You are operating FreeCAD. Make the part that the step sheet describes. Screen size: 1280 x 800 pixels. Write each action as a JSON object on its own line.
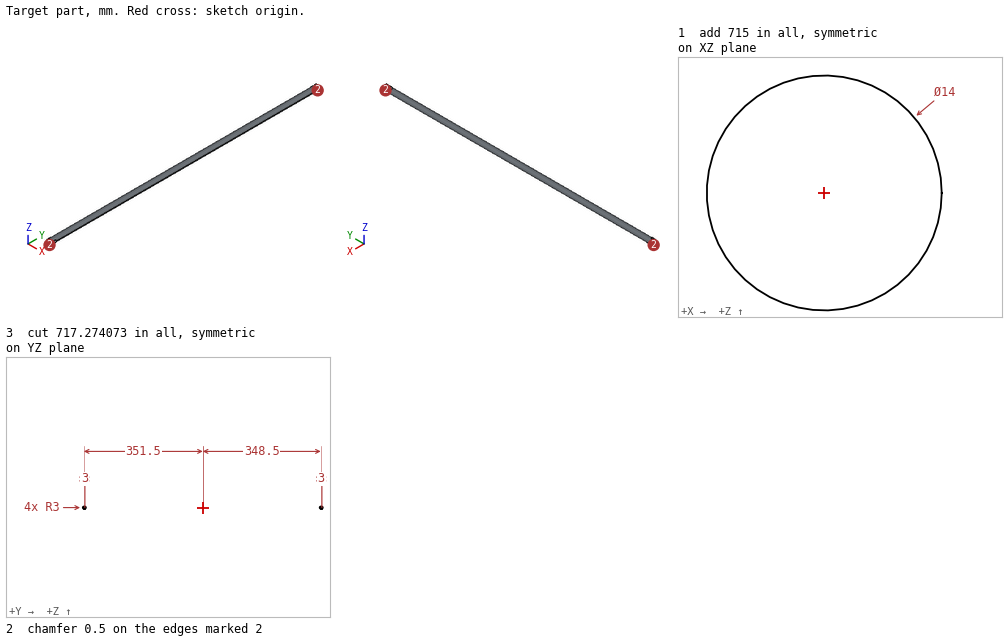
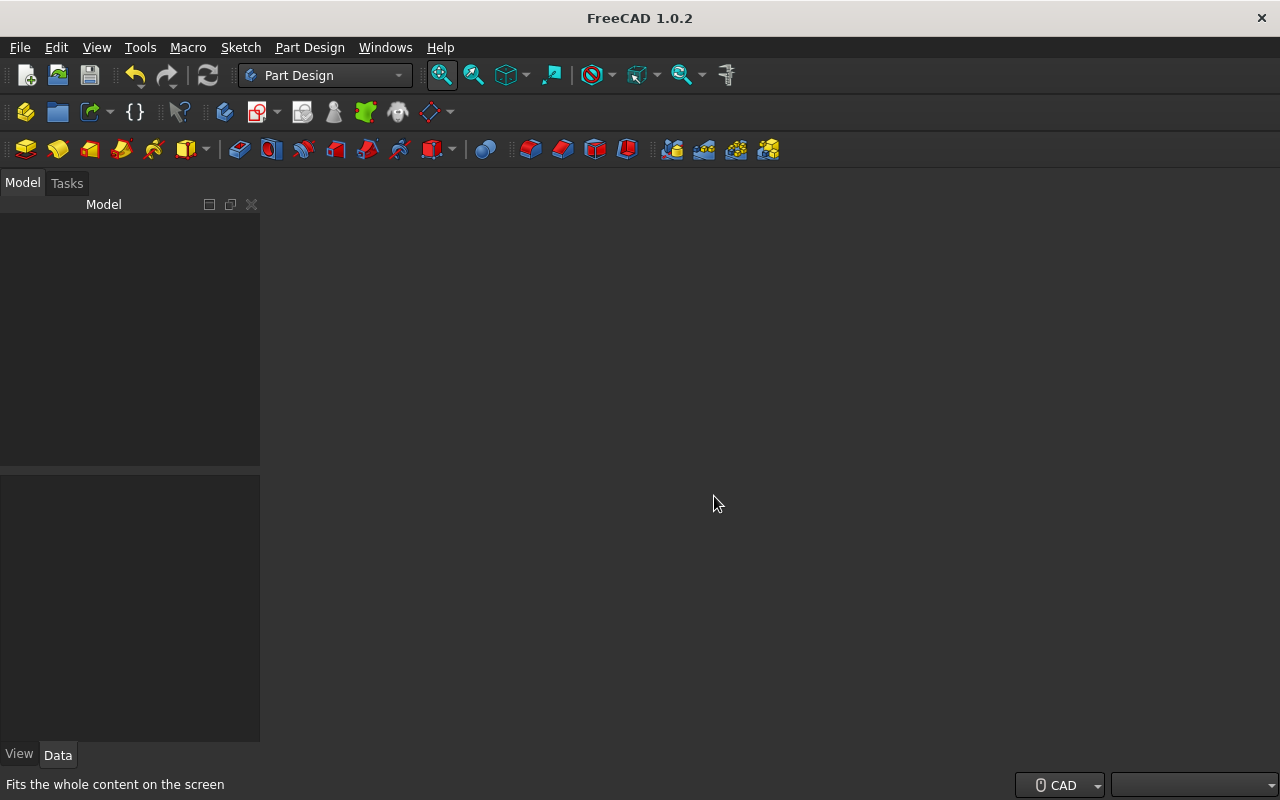
{"action": "left_click", "coordinate": [26, 76]}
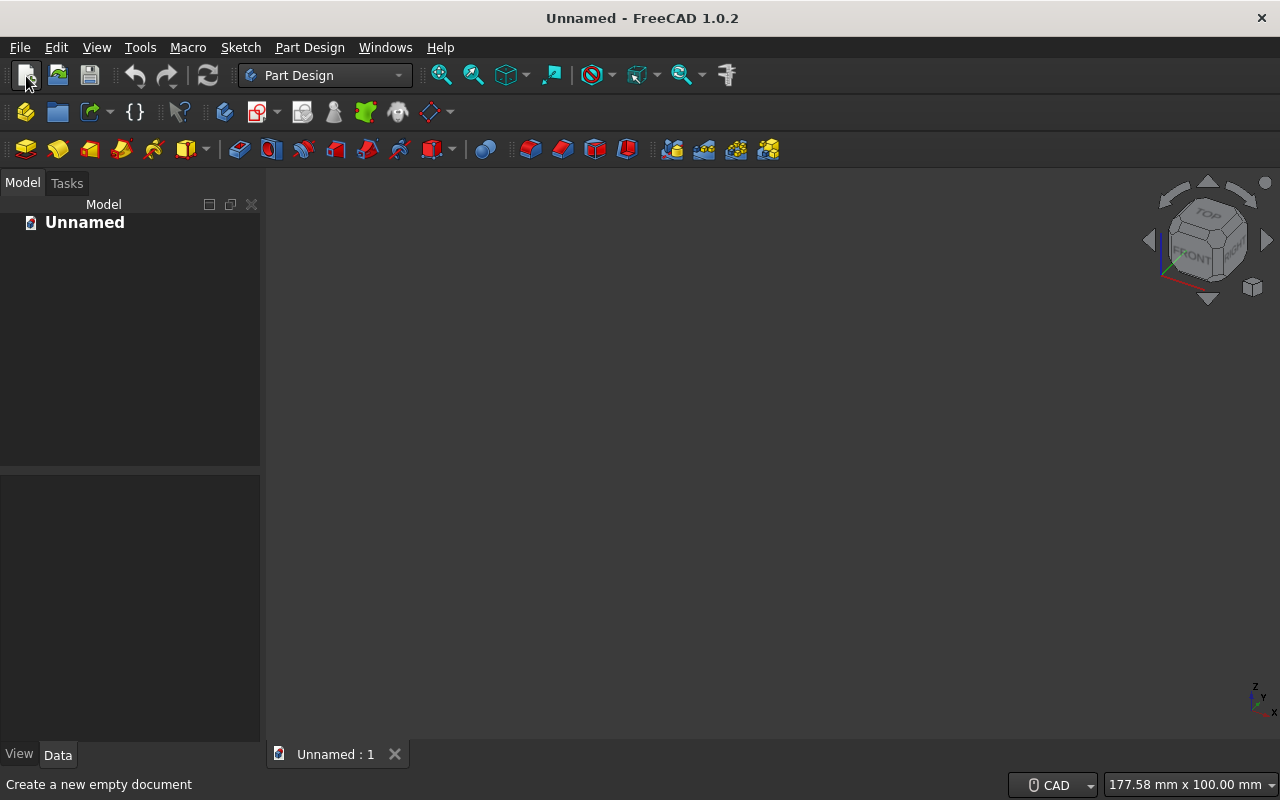
{"action": "left_click", "coordinate": [258, 112]}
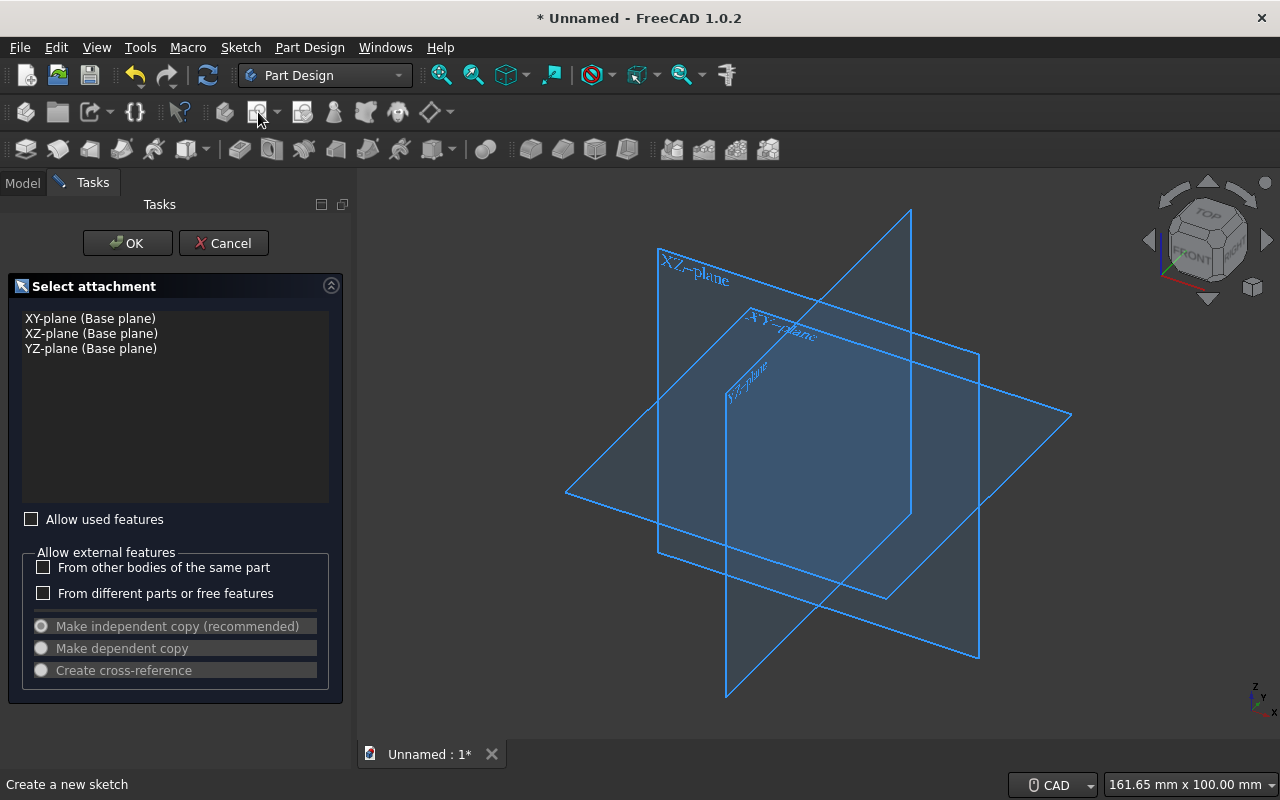
{"action": "left_click", "coordinate": [82, 334]}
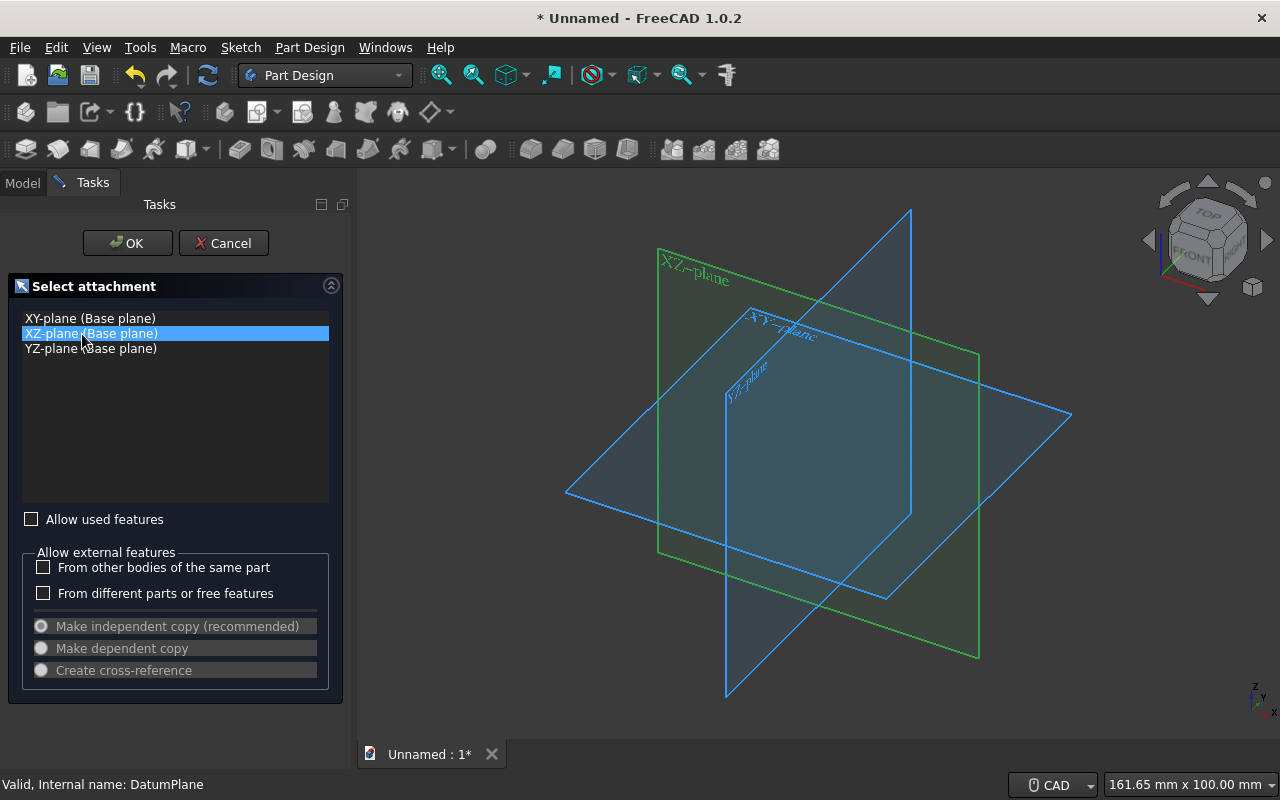
{"action": "left_click", "coordinate": [128, 243]}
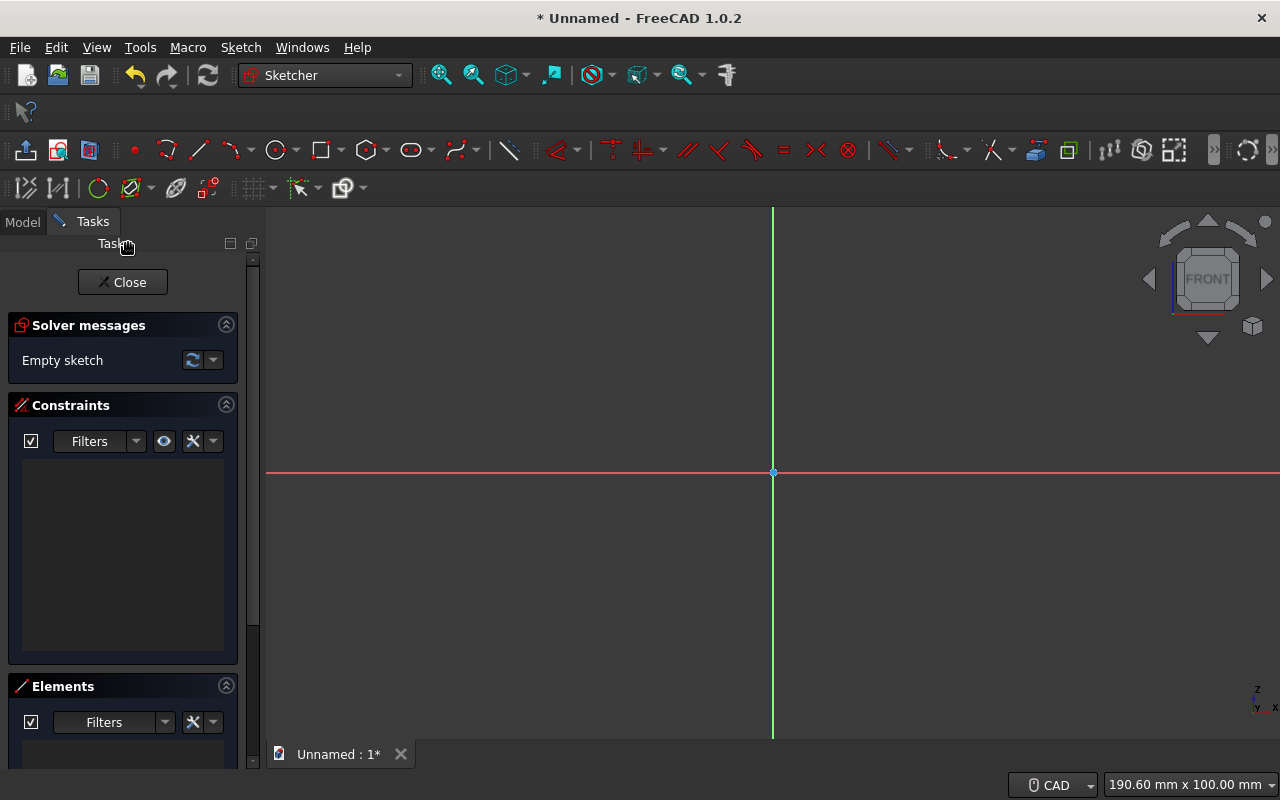
{"action": "scroll", "coordinate": [790, 473], "scroll_direction": "up", "scroll_amount": 8}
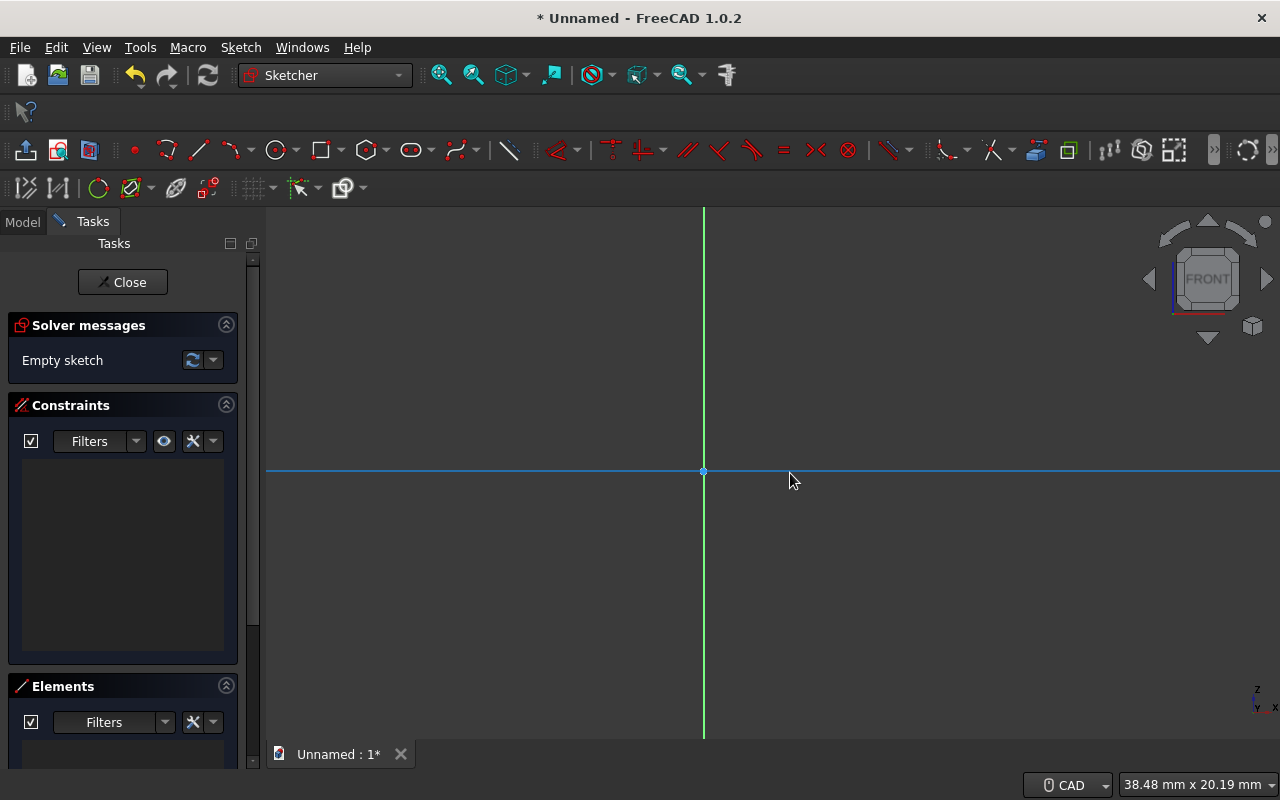
{"action": "left_click", "coordinate": [276, 150]}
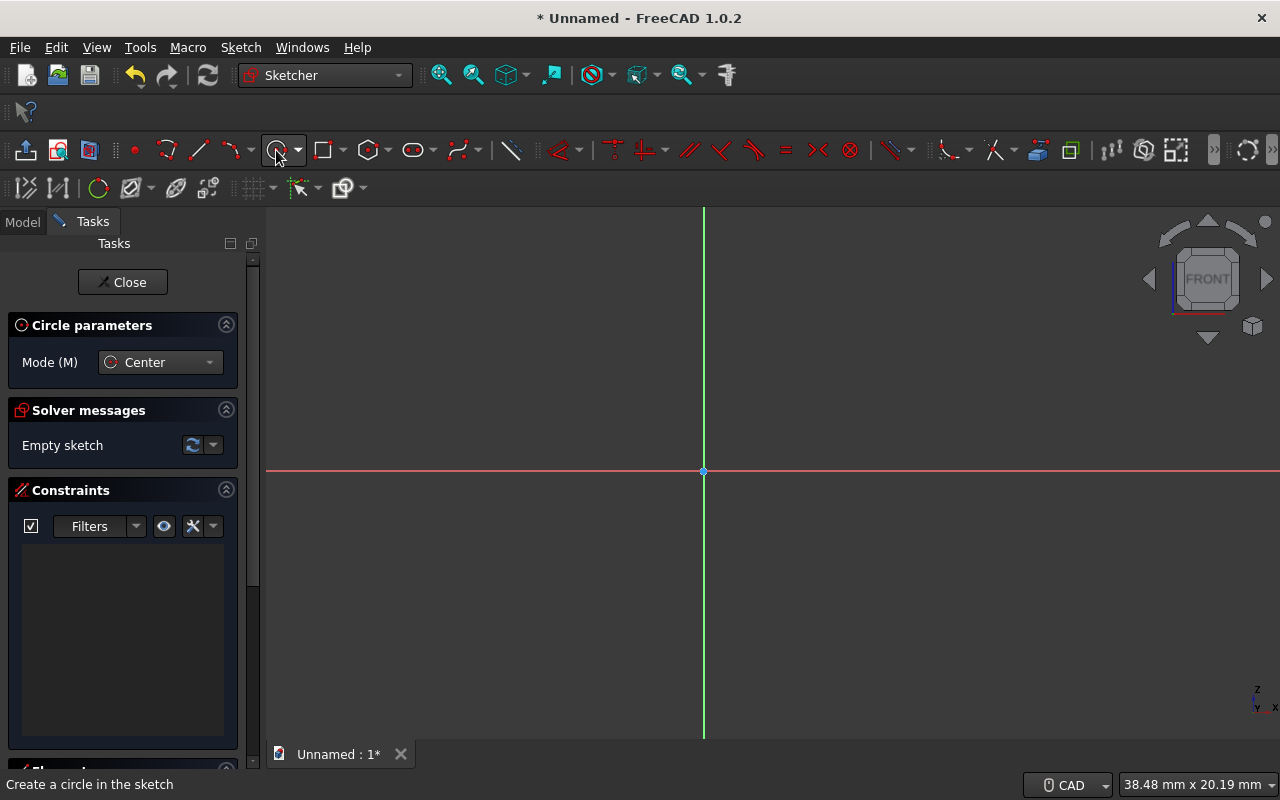
{"action": "left_click", "coordinate": [704, 471]}
{"action": "left_click", "coordinate": [834, 341]}
{"action": "key", "text": "Escape"}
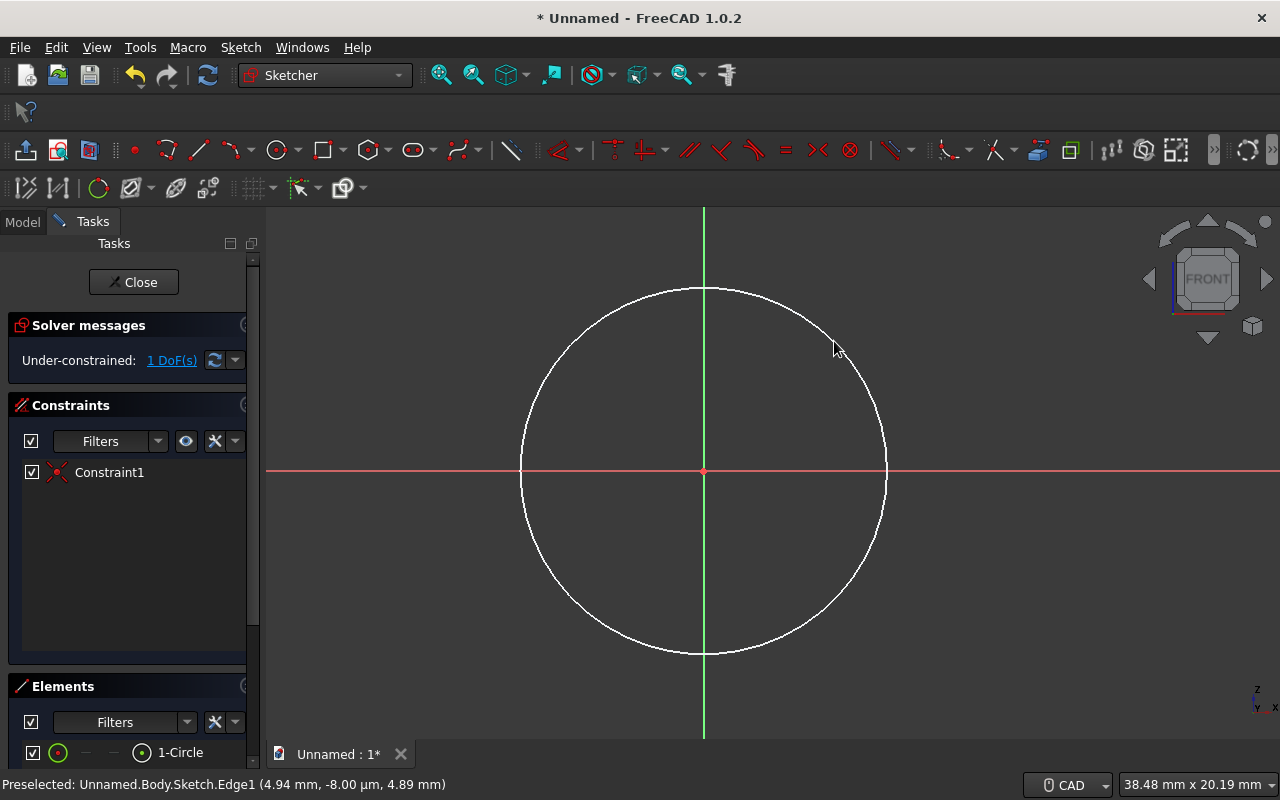
{"action": "left_click", "coordinate": [833, 341]}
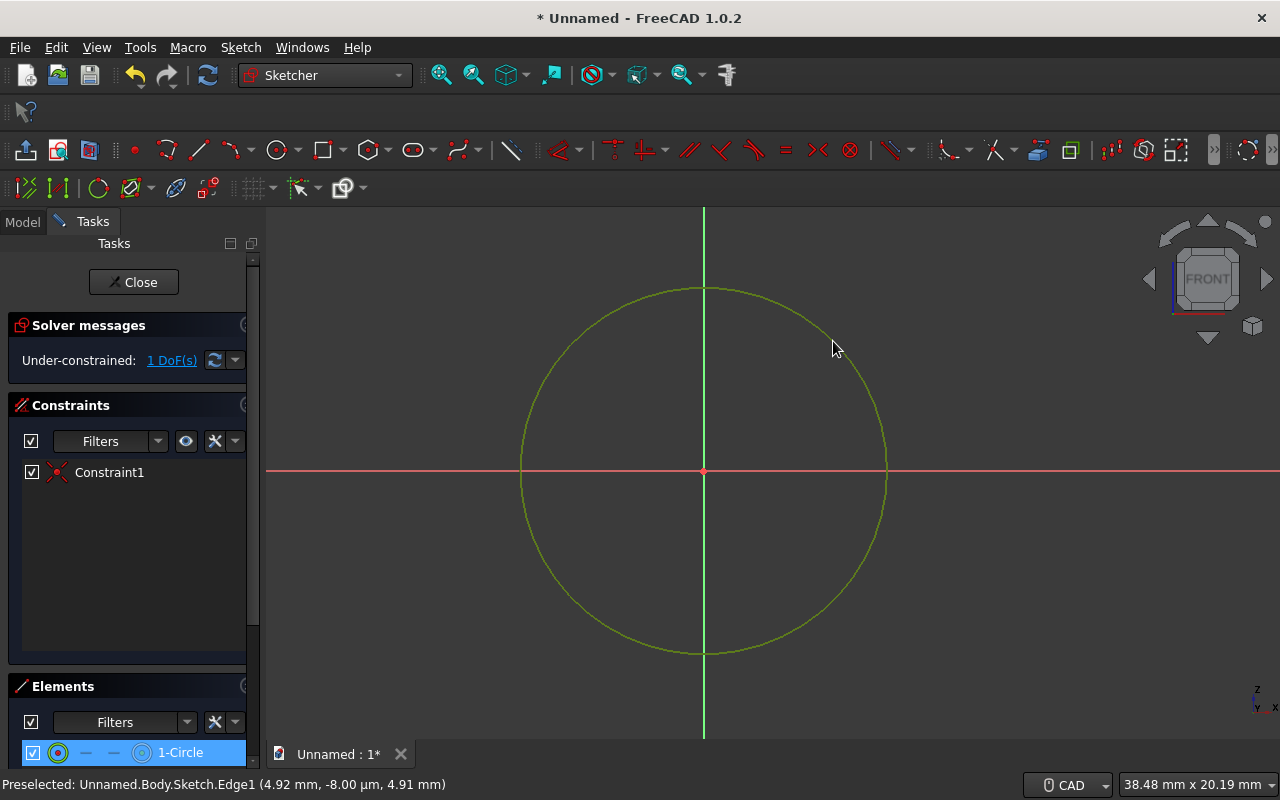
{"action": "key", "text": "k o"}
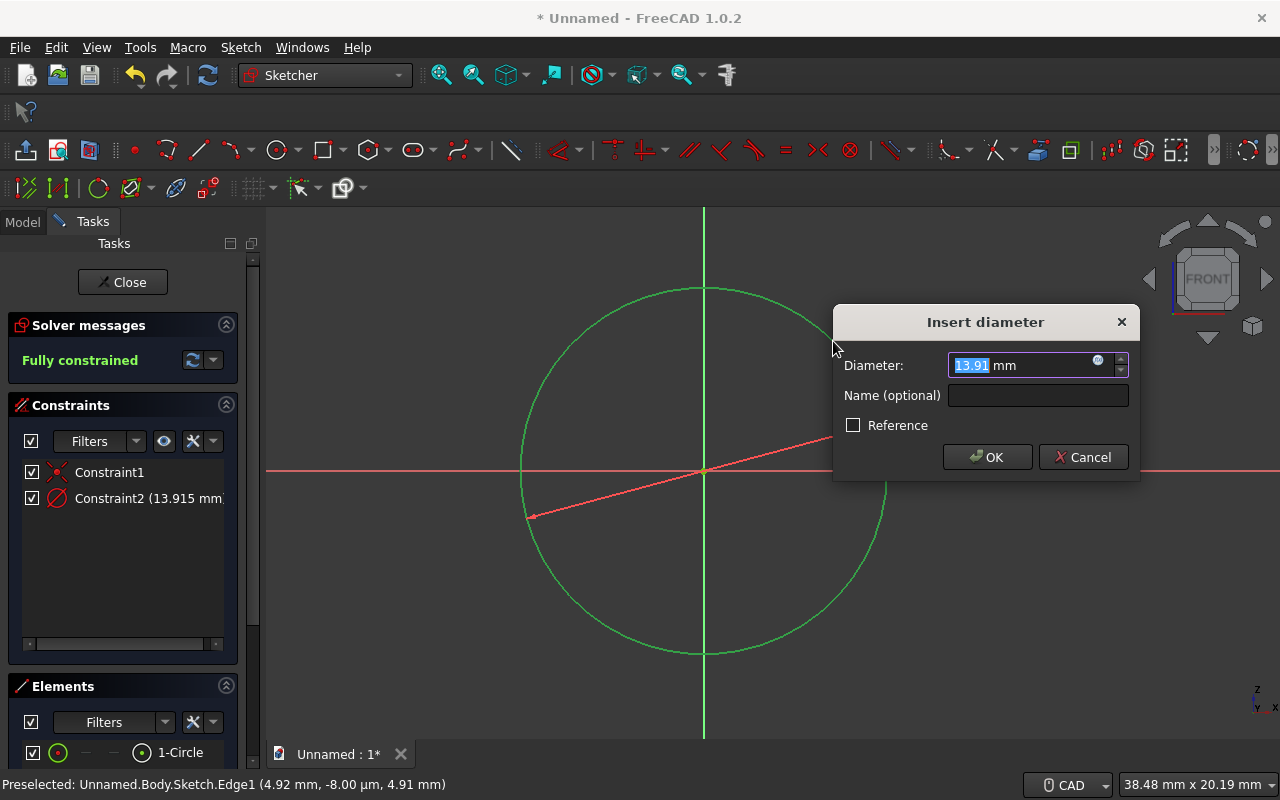
{"action": "type", "text": "14"}
{"action": "key", "text": "Return"}